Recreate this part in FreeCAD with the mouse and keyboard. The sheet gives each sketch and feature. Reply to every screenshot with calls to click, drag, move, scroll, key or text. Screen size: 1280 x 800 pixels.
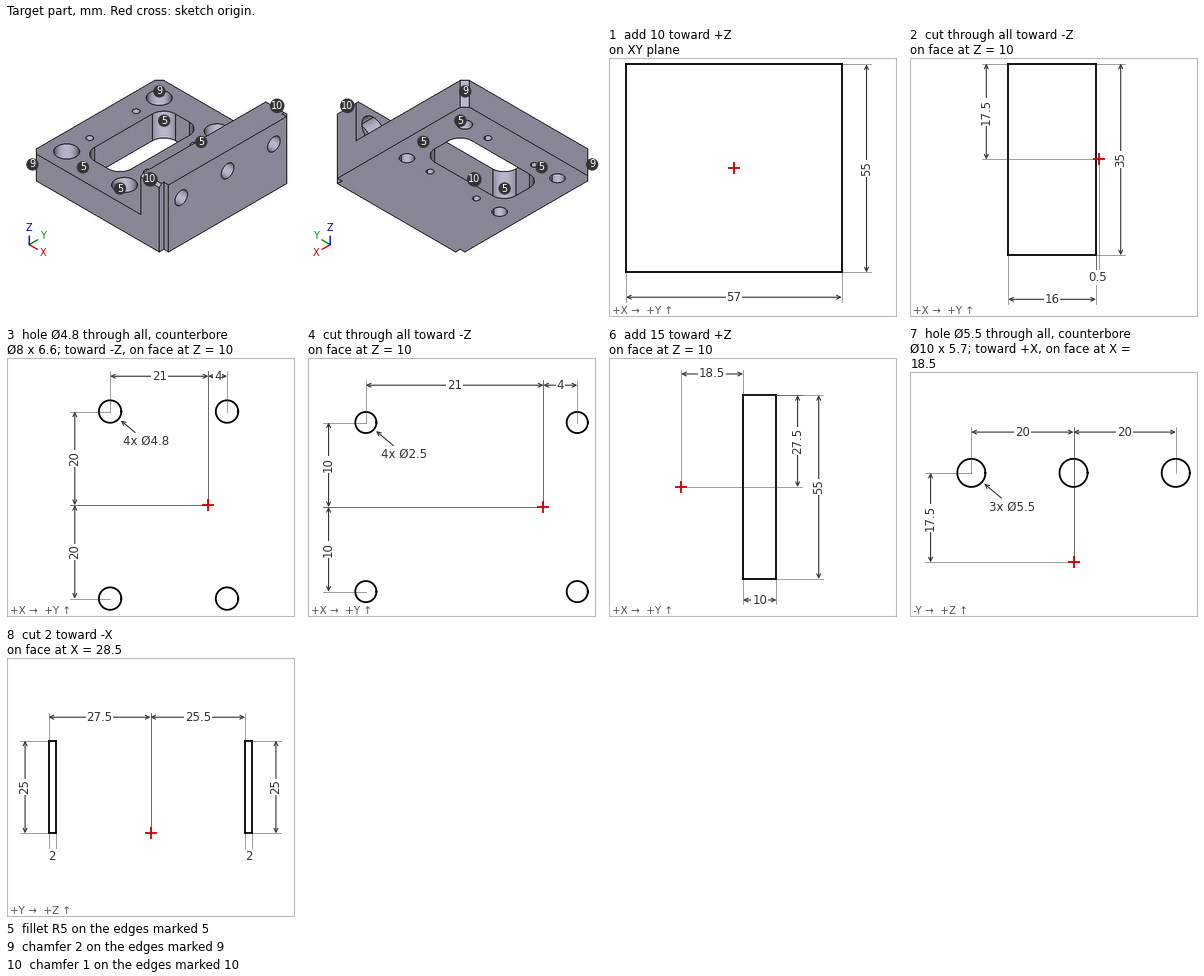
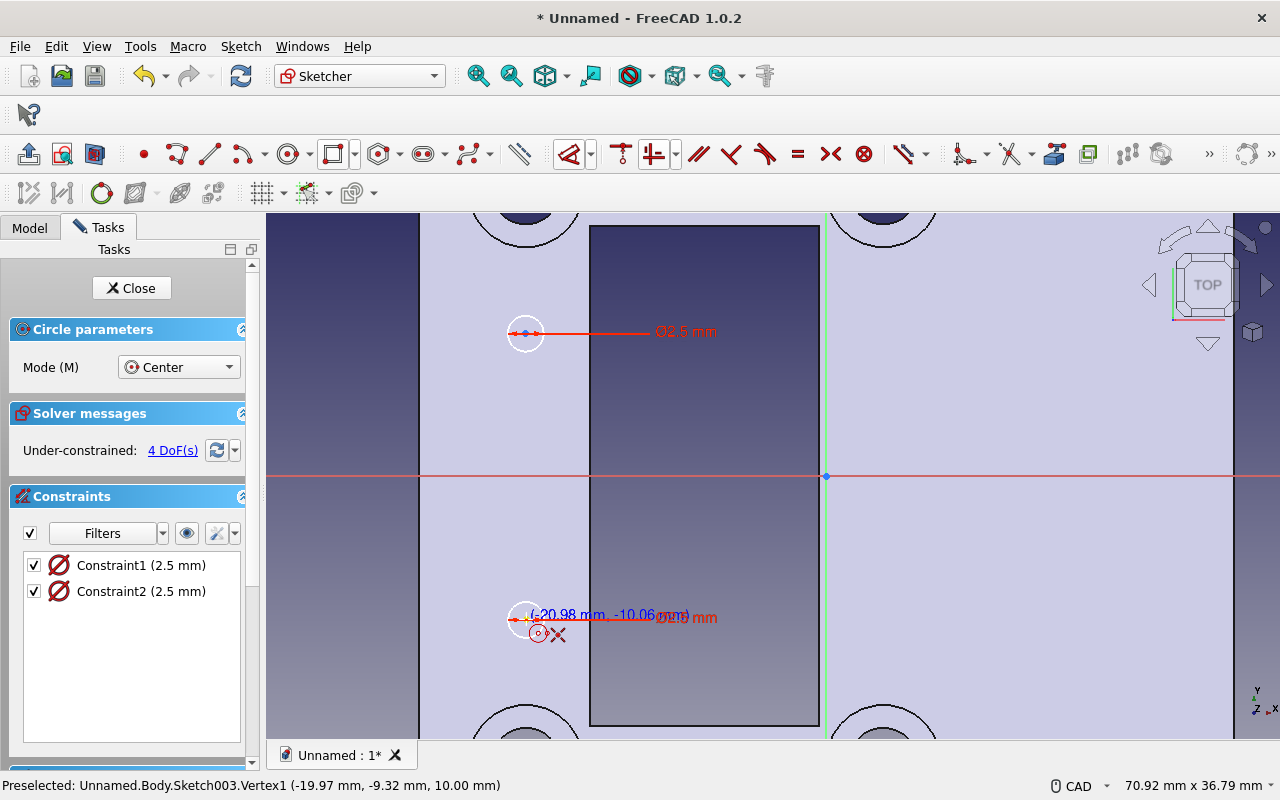
scroll(883, 333, up, 2)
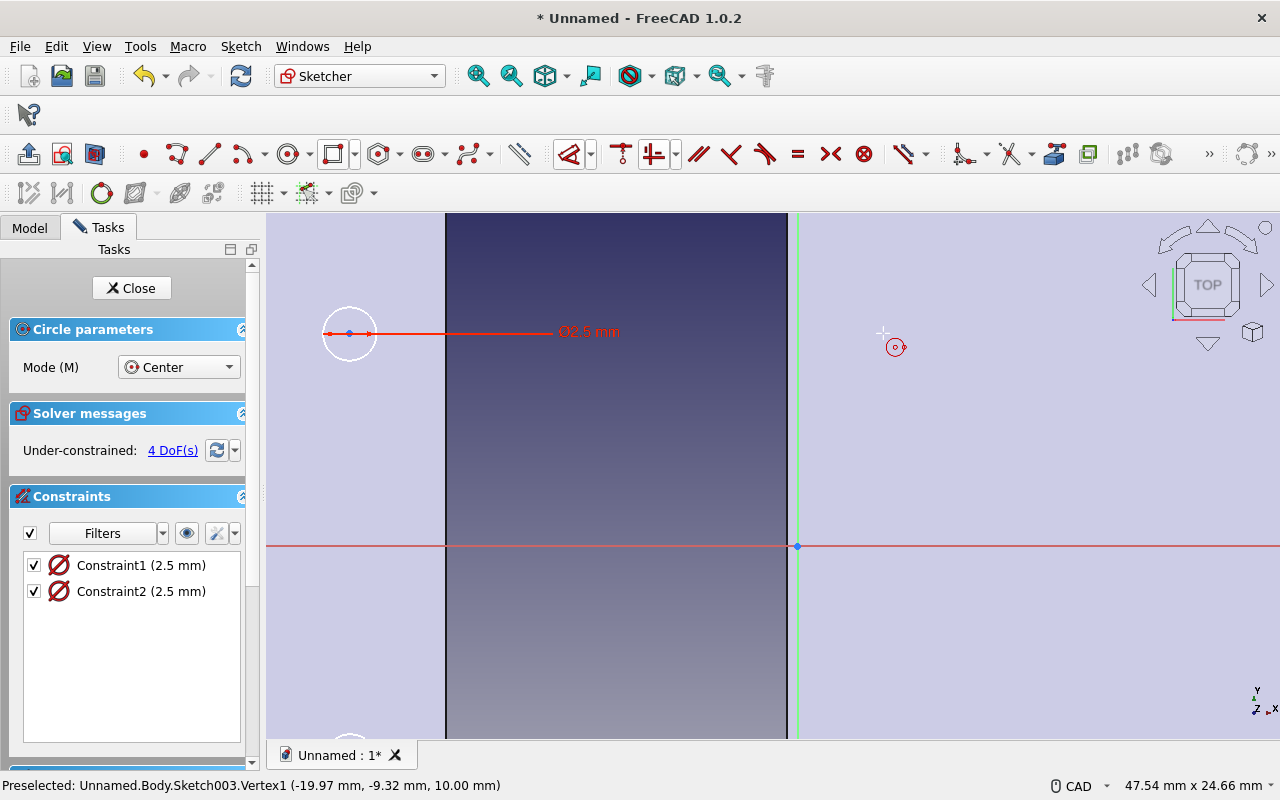
click(883, 333)
move(902, 314)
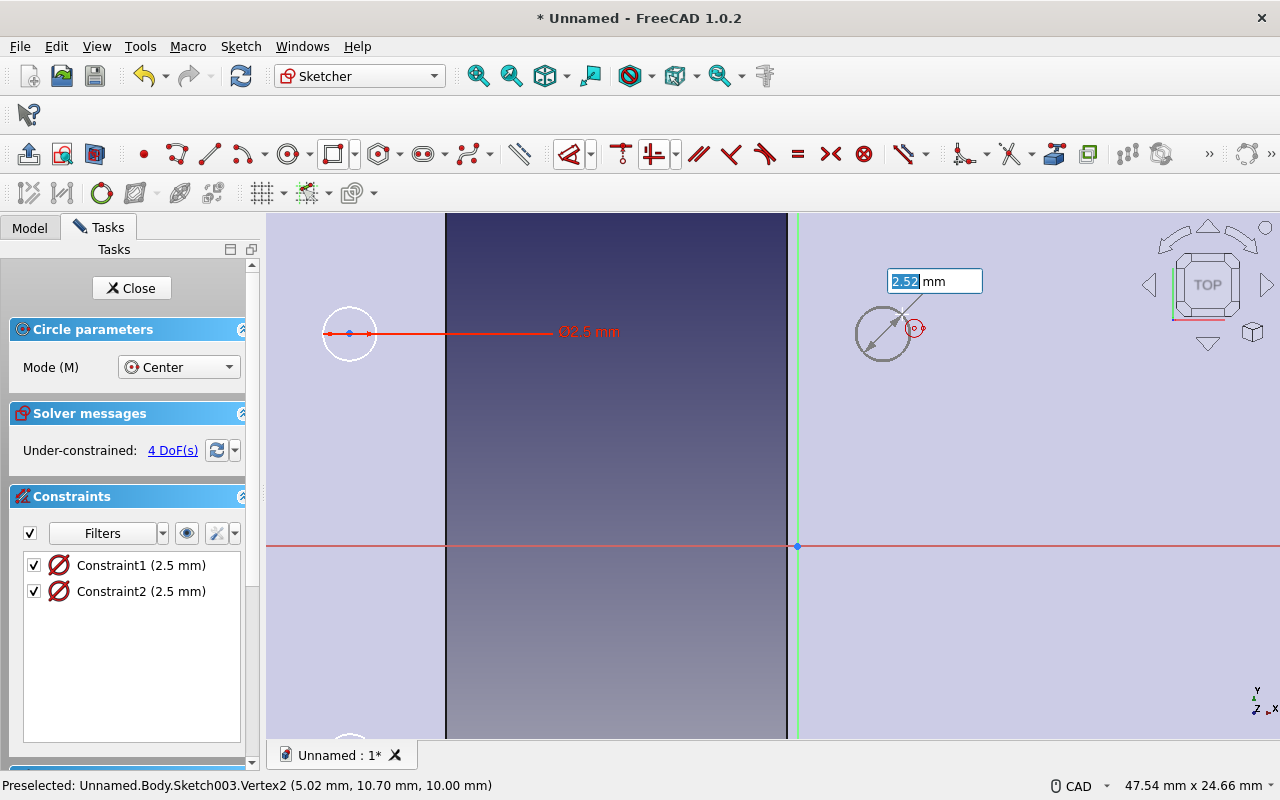
text(2.5)
key(Return)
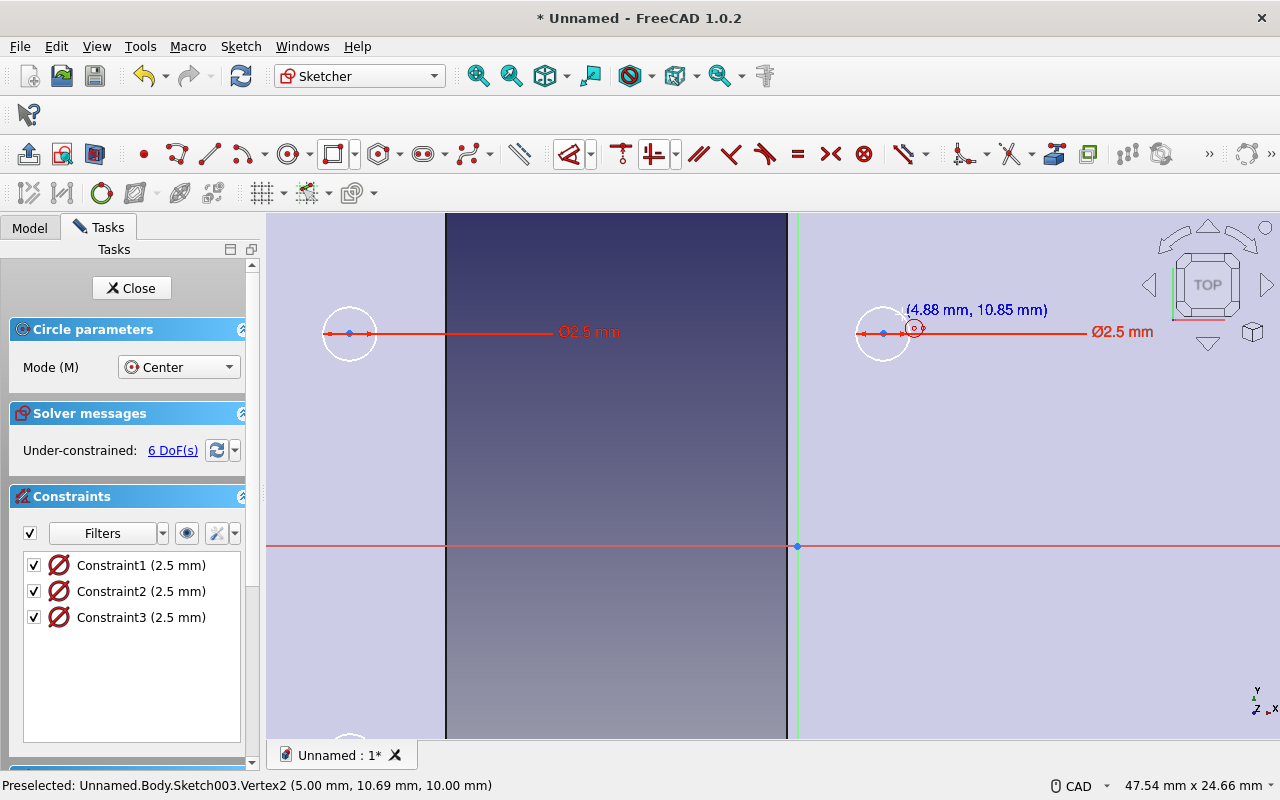
scroll(883, 333, down, 2)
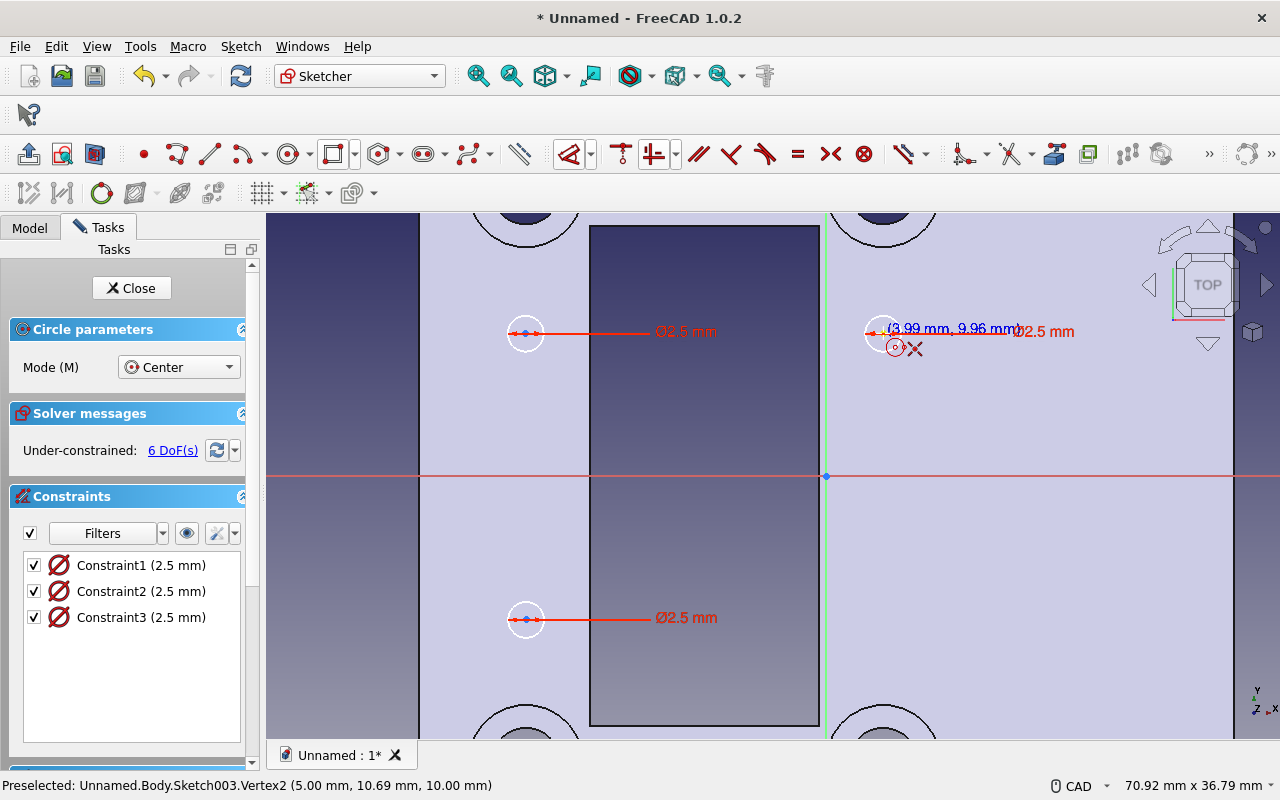
scroll(883, 619, up, 2)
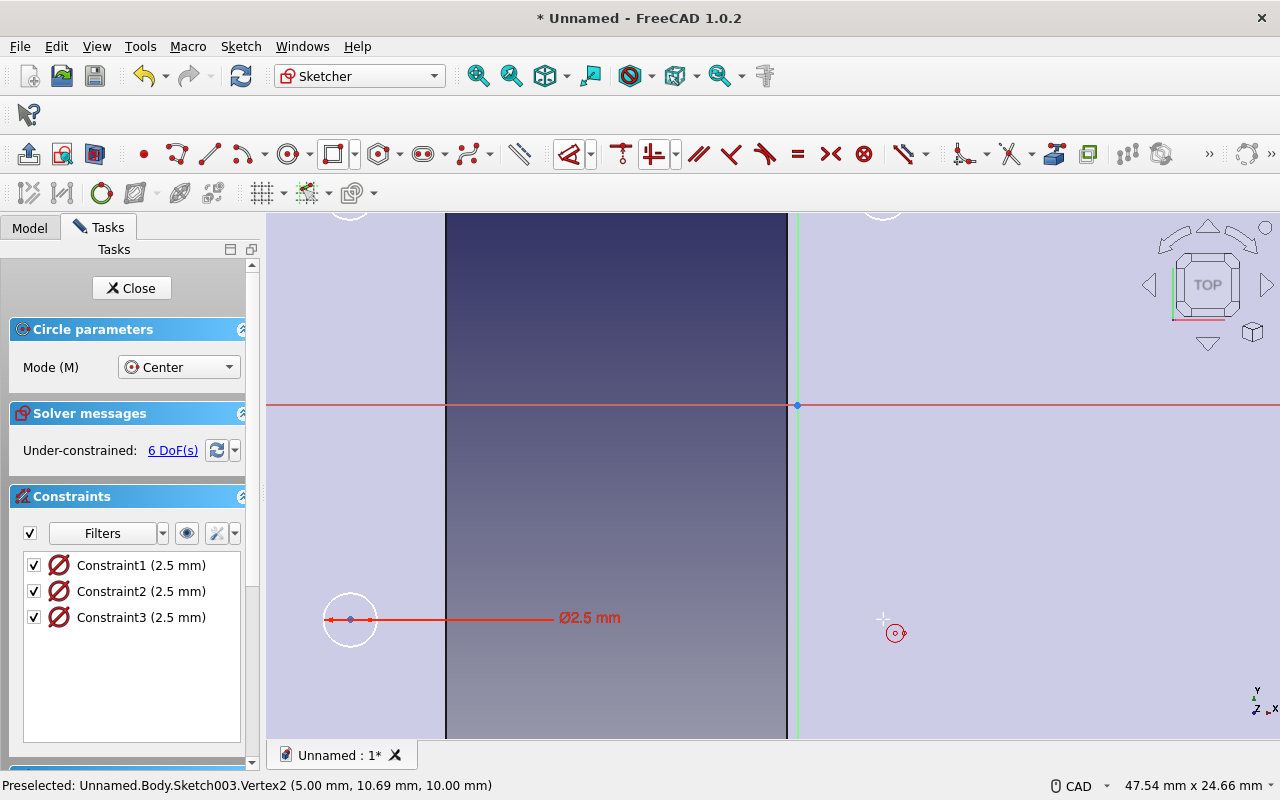
click(883, 619)
move(902, 600)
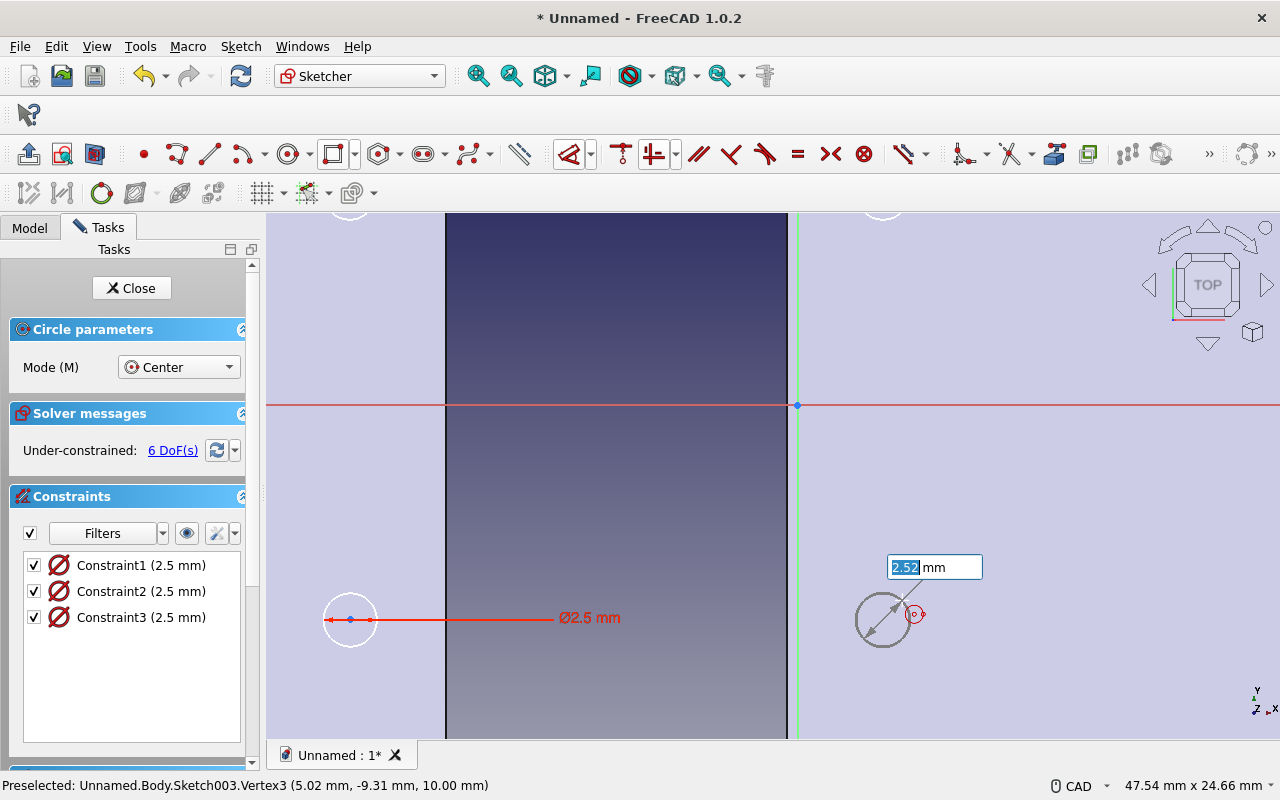
text(2.5)
key(Return)
key(Escape)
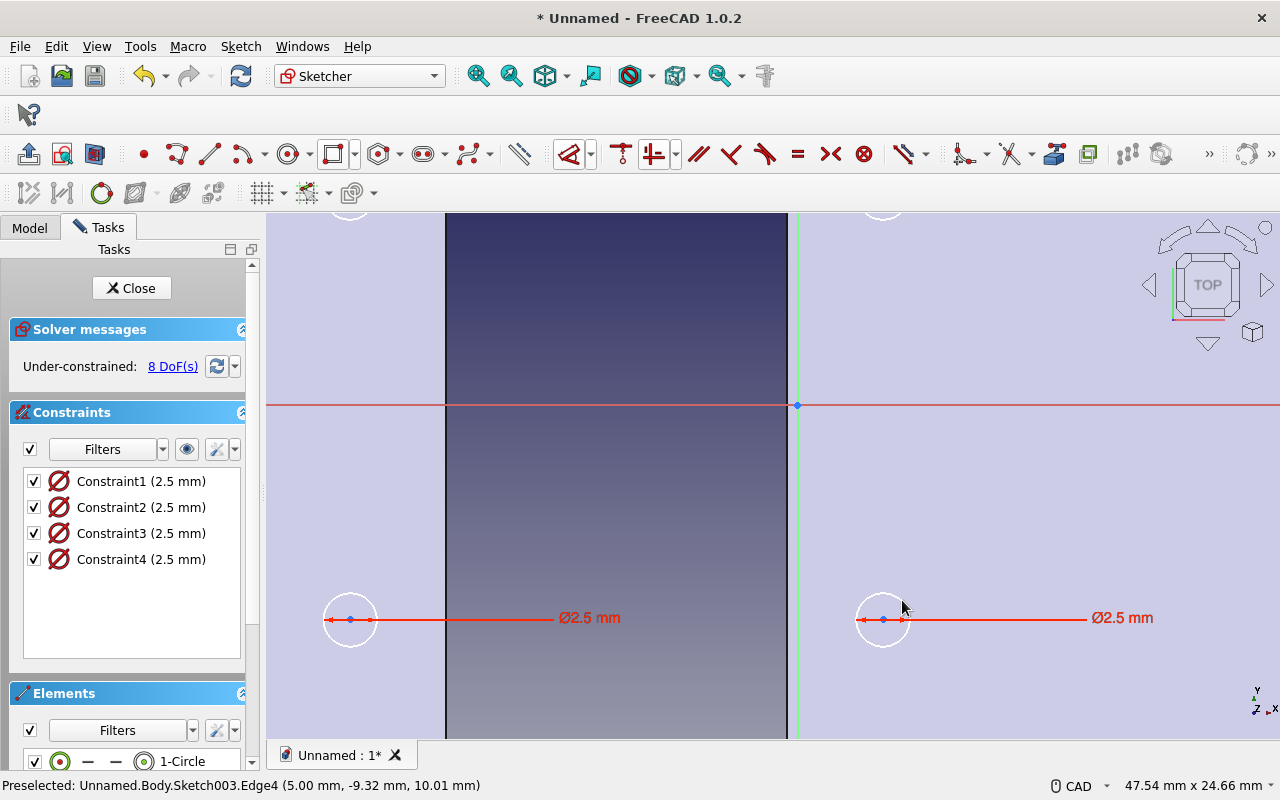
scroll(883, 619, down, 2)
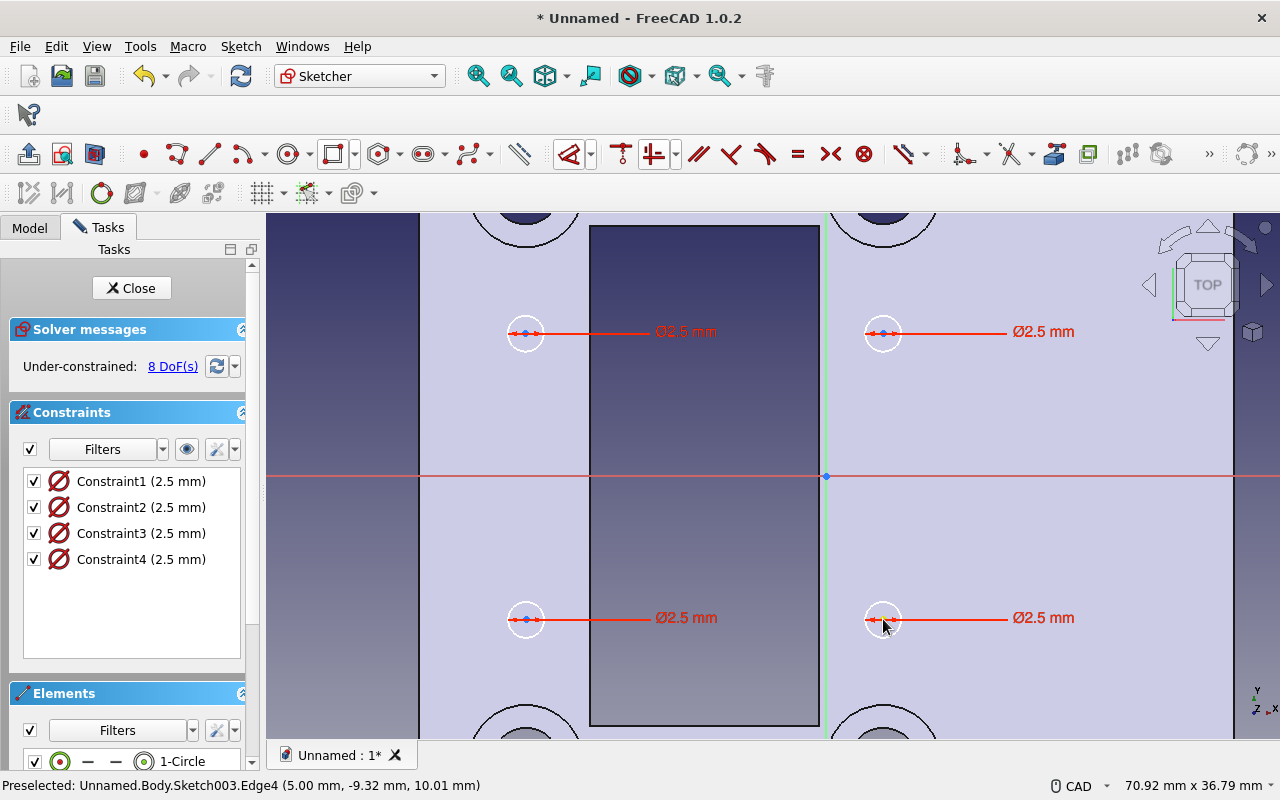
click(526, 334)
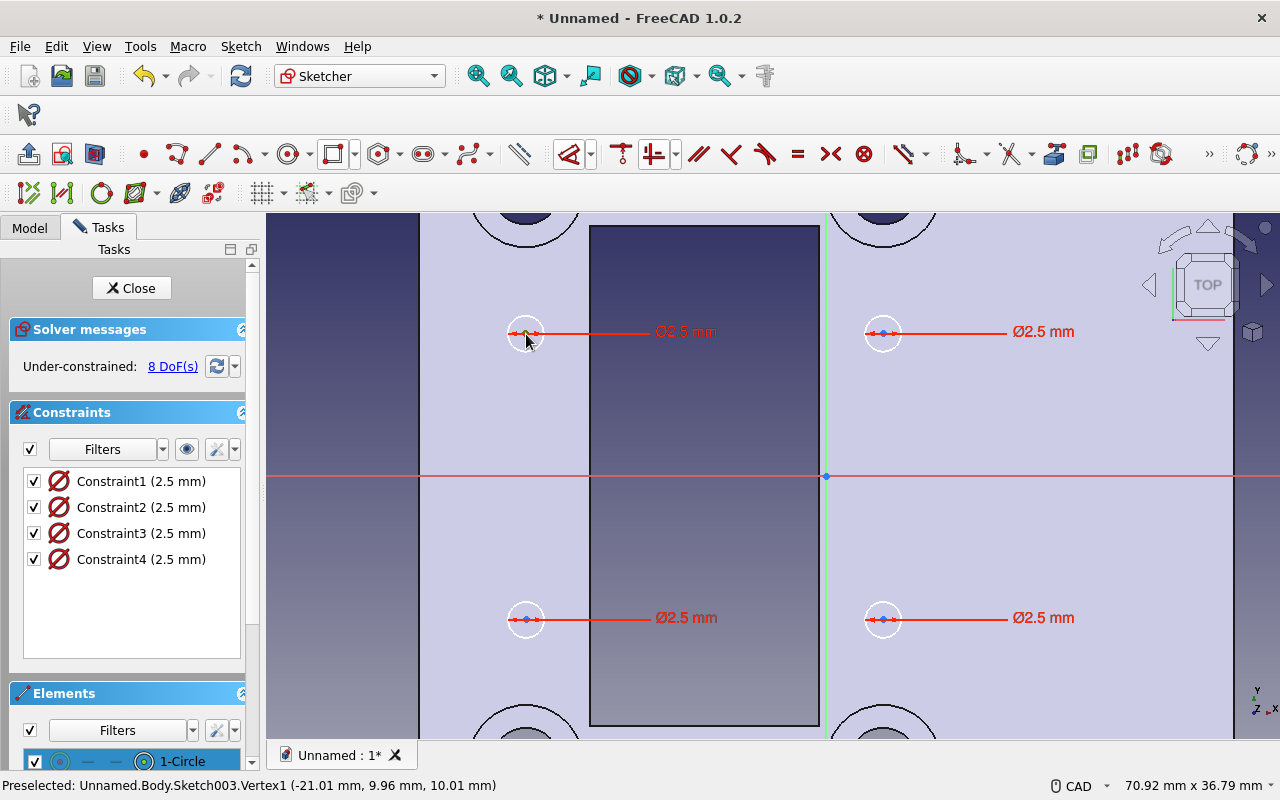
click(526, 620)